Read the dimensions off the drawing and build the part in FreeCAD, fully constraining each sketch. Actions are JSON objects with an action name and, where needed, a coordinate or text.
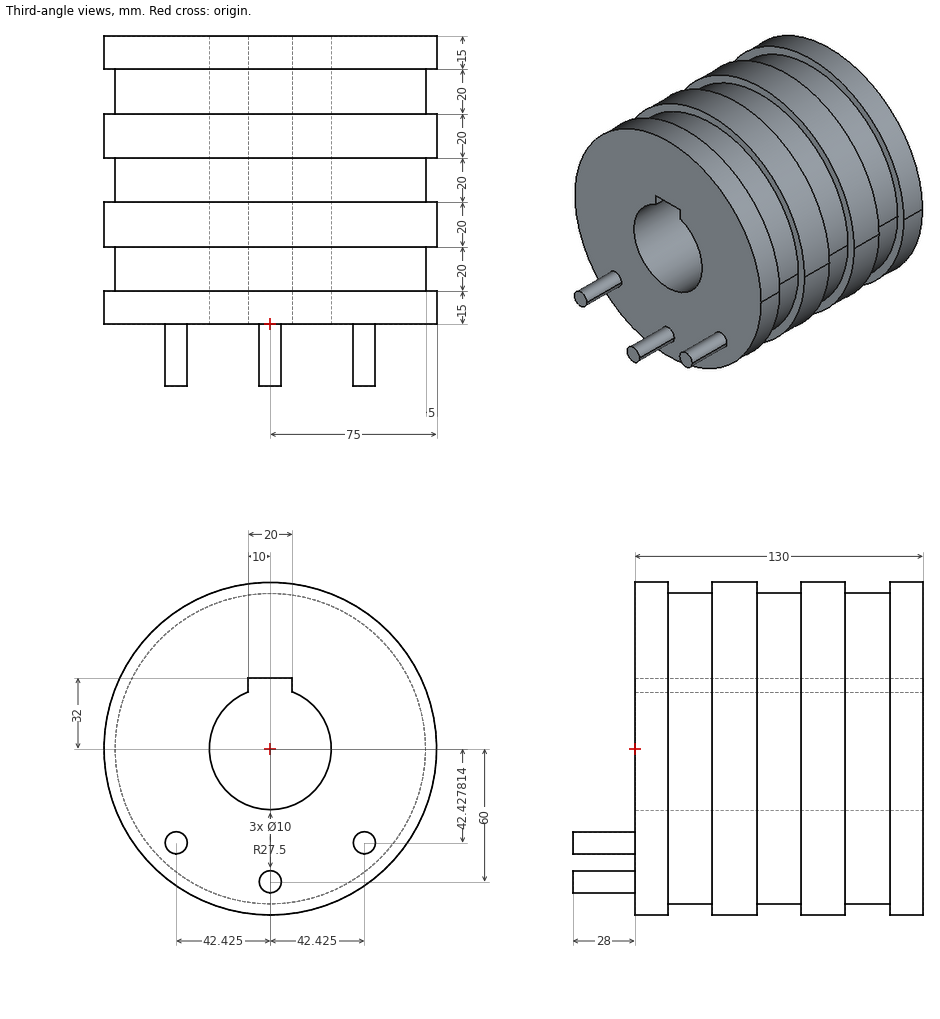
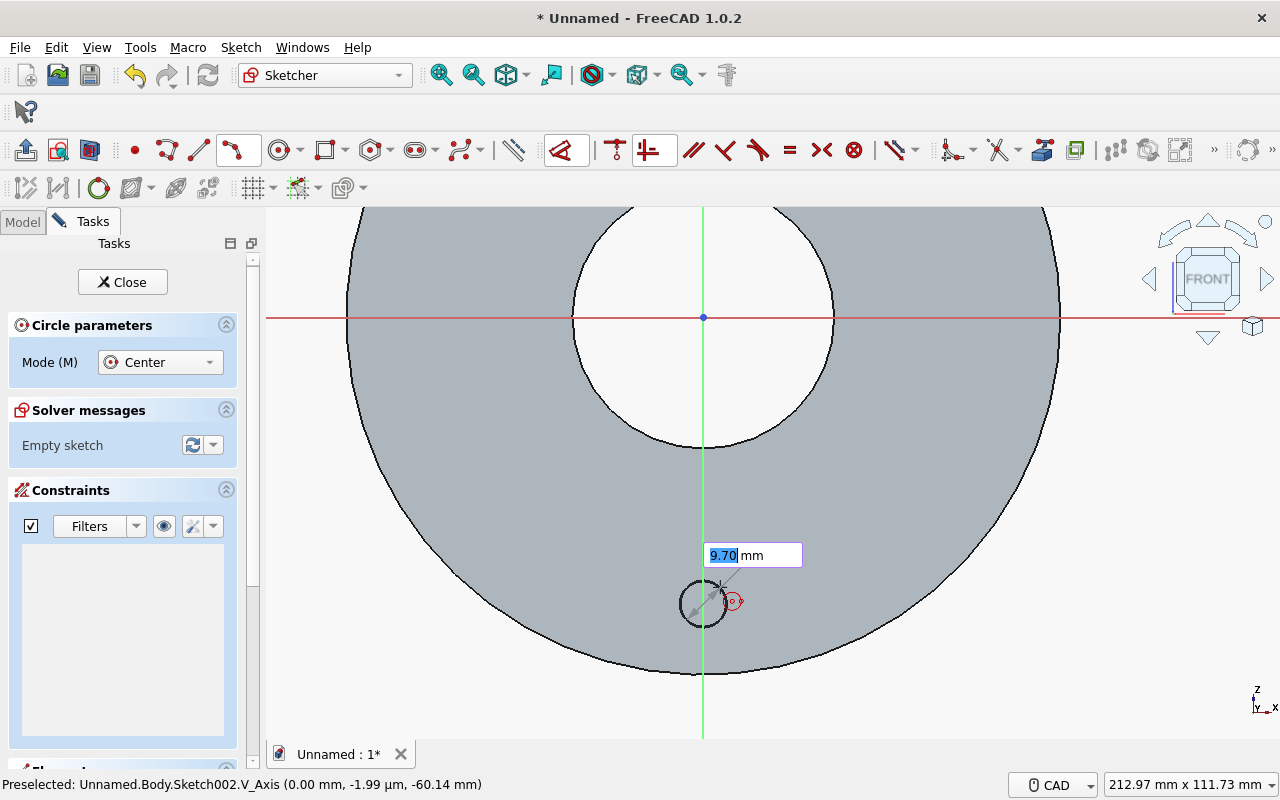
{"action": "type", "text": "10"}
{"action": "key", "text": "Return"}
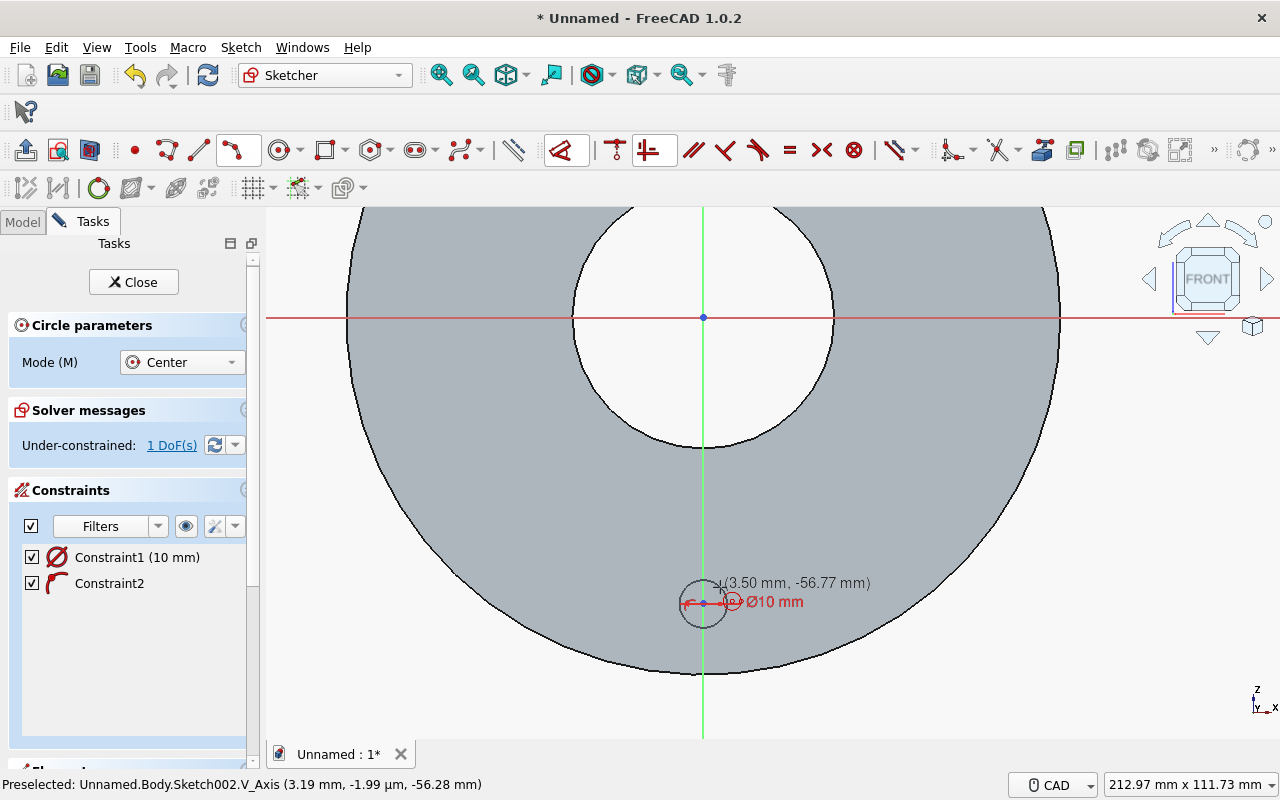
{"action": "left_click", "coordinate": [905, 520]}
{"action": "mouse_move", "coordinate": [922, 503]}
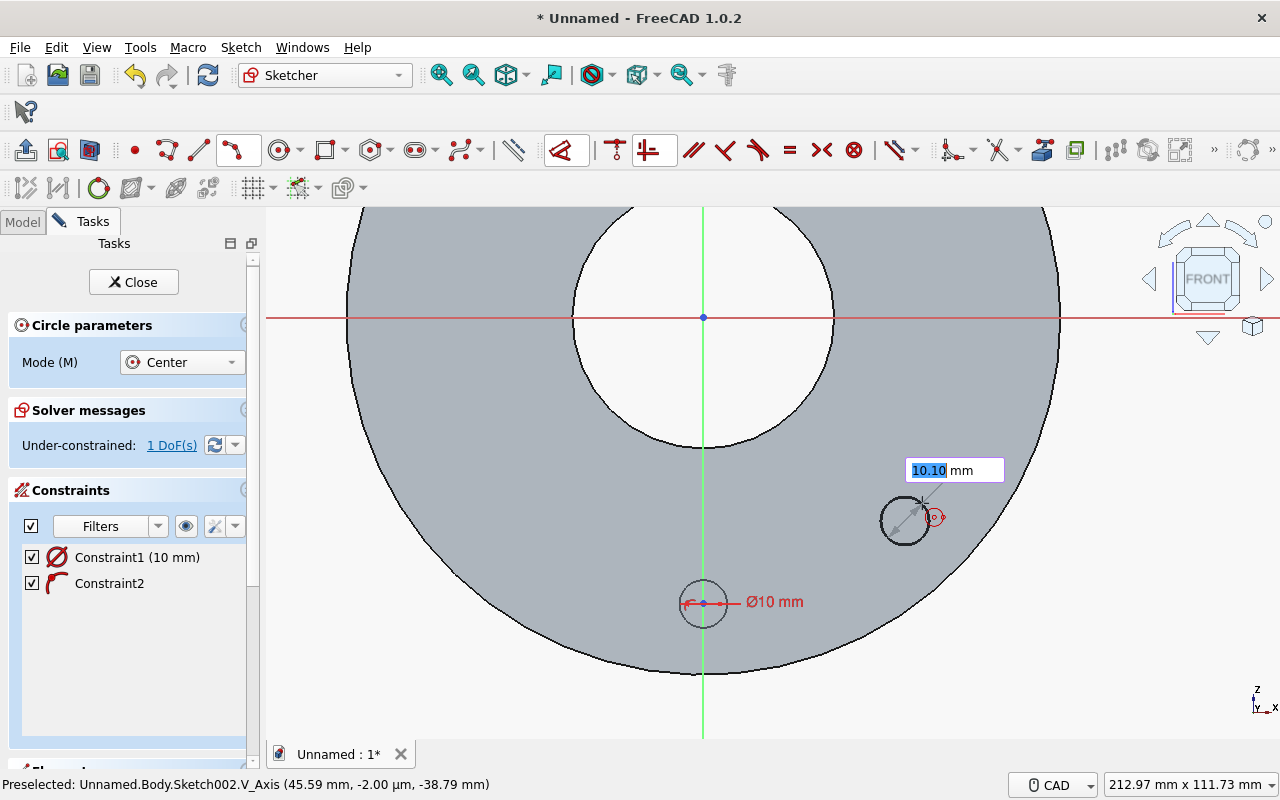
{"action": "type", "text": "10"}
{"action": "key", "text": "Return"}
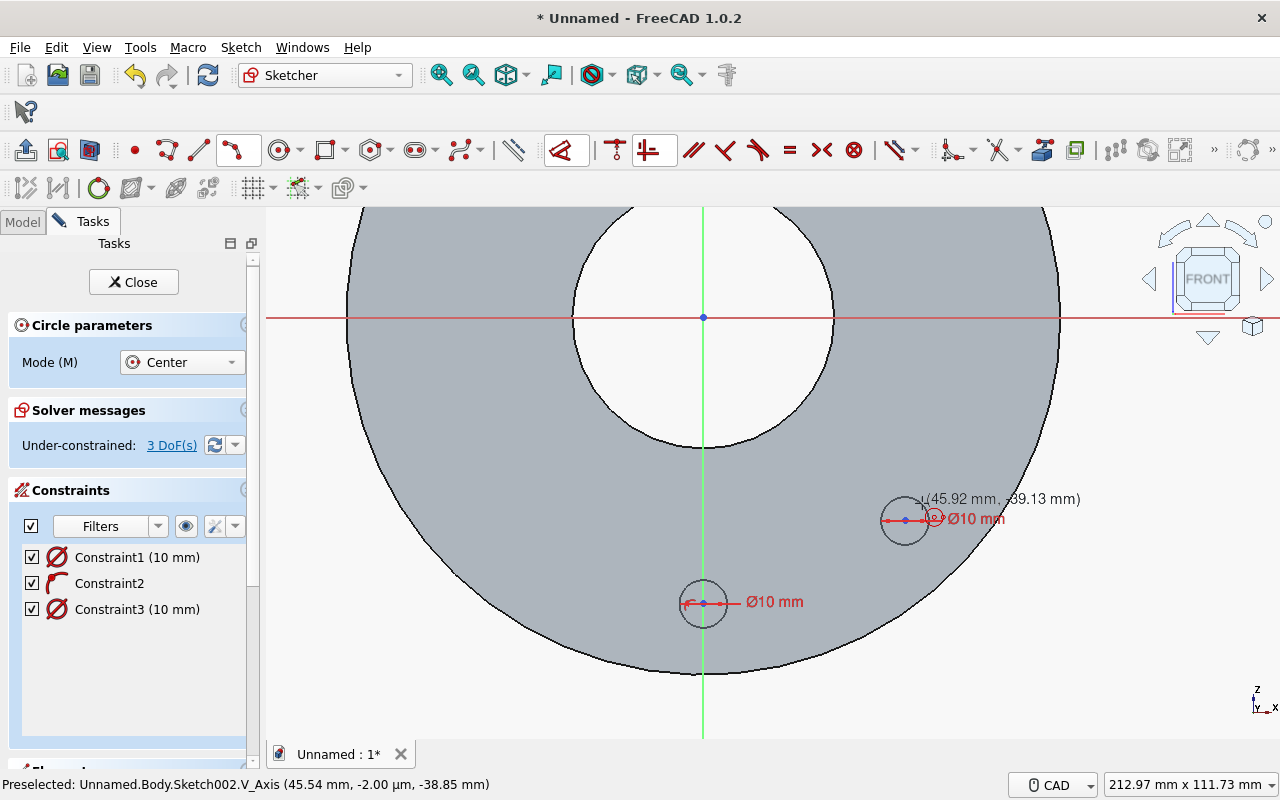
{"action": "left_click", "coordinate": [501, 520]}
{"action": "mouse_move", "coordinate": [518, 503]}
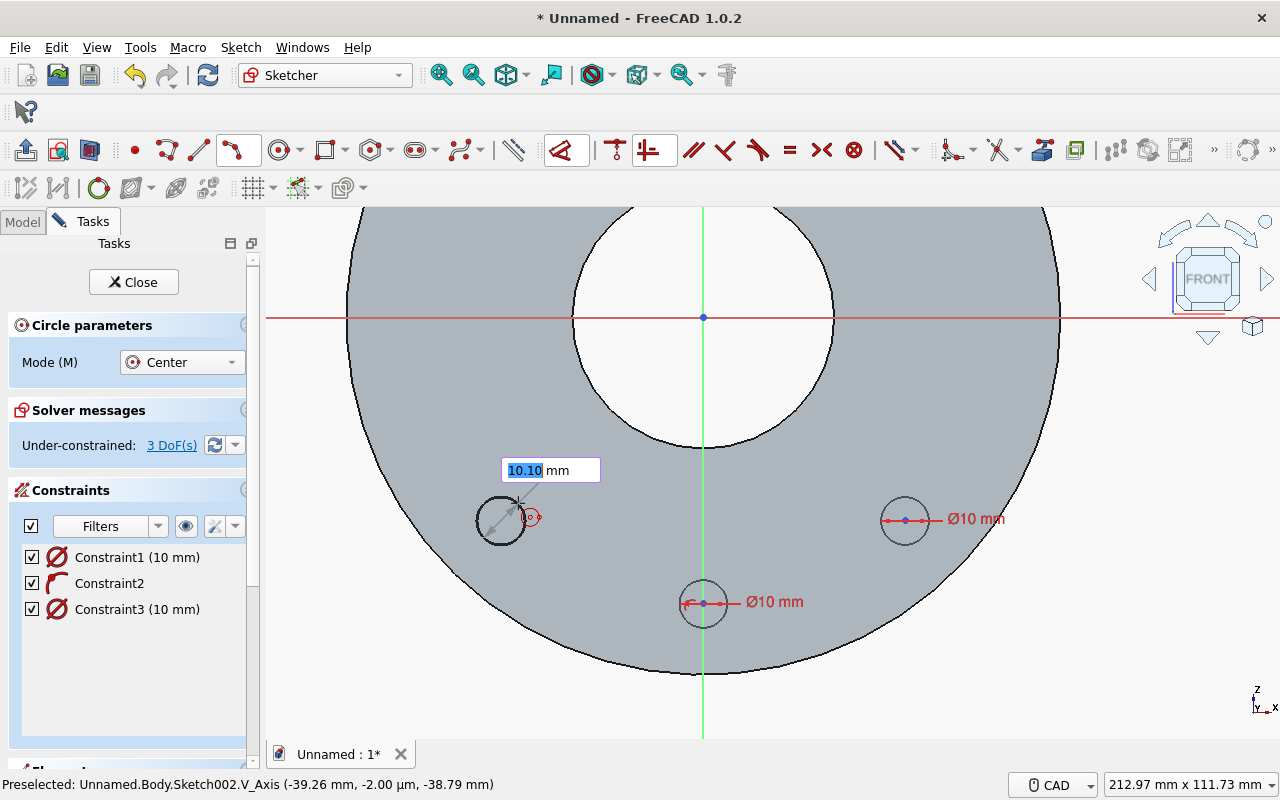
{"action": "type", "text": "10"}
{"action": "key", "text": "Return"}
{"action": "key", "text": "Escape"}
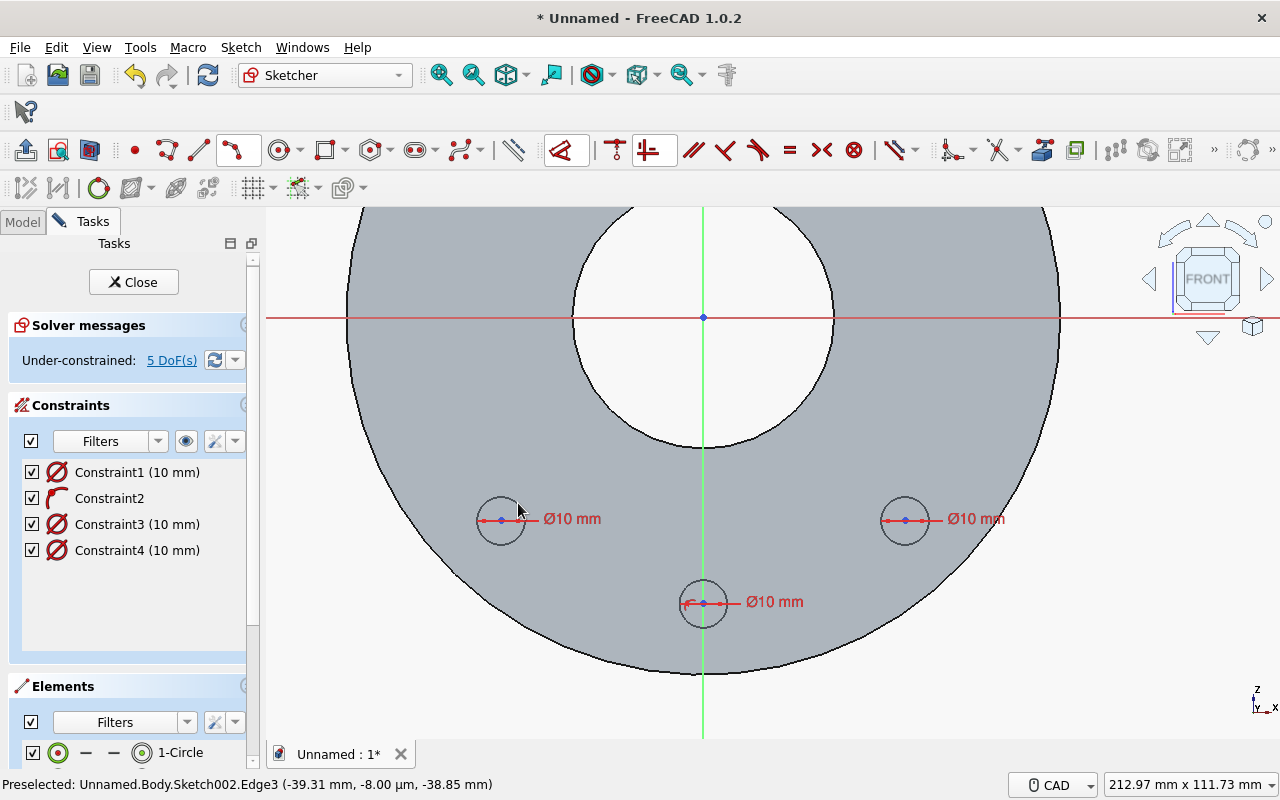
{"action": "left_click", "coordinate": [905, 521]}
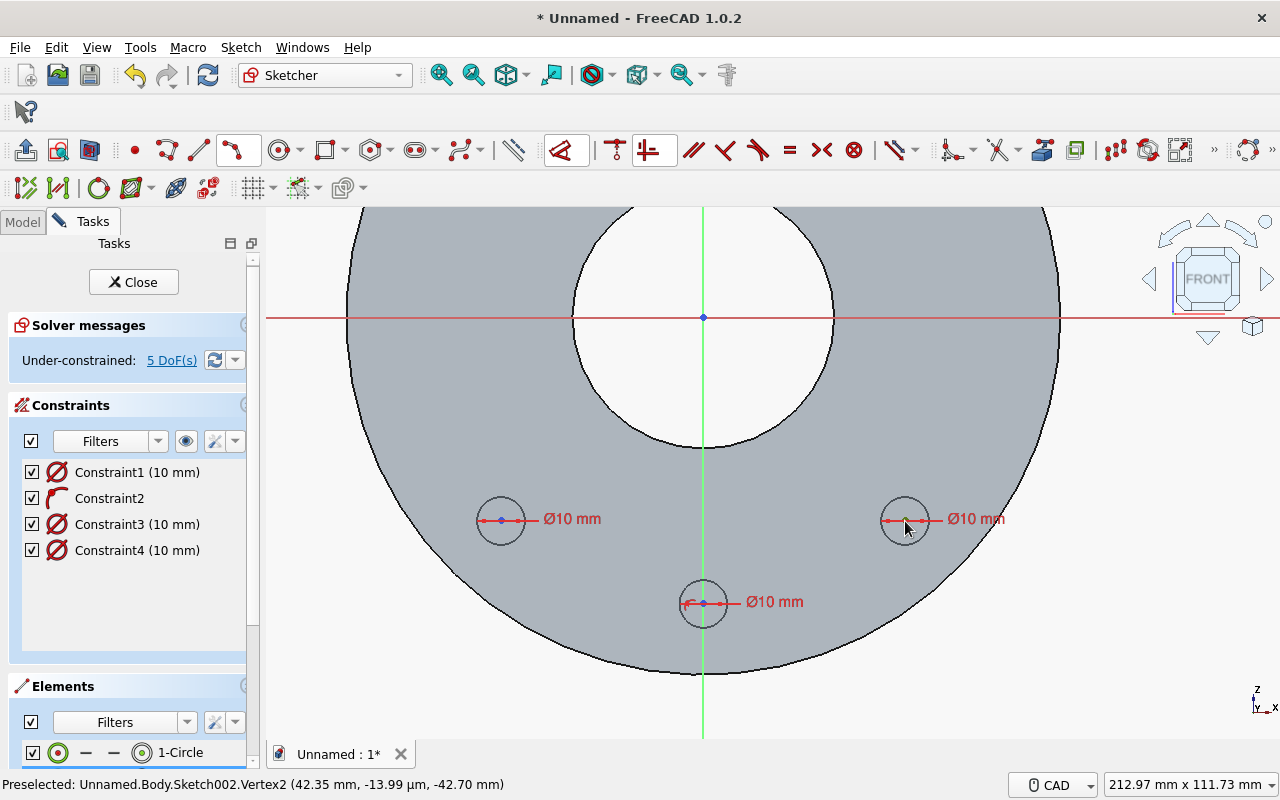
{"action": "left_click", "coordinate": [501, 521]}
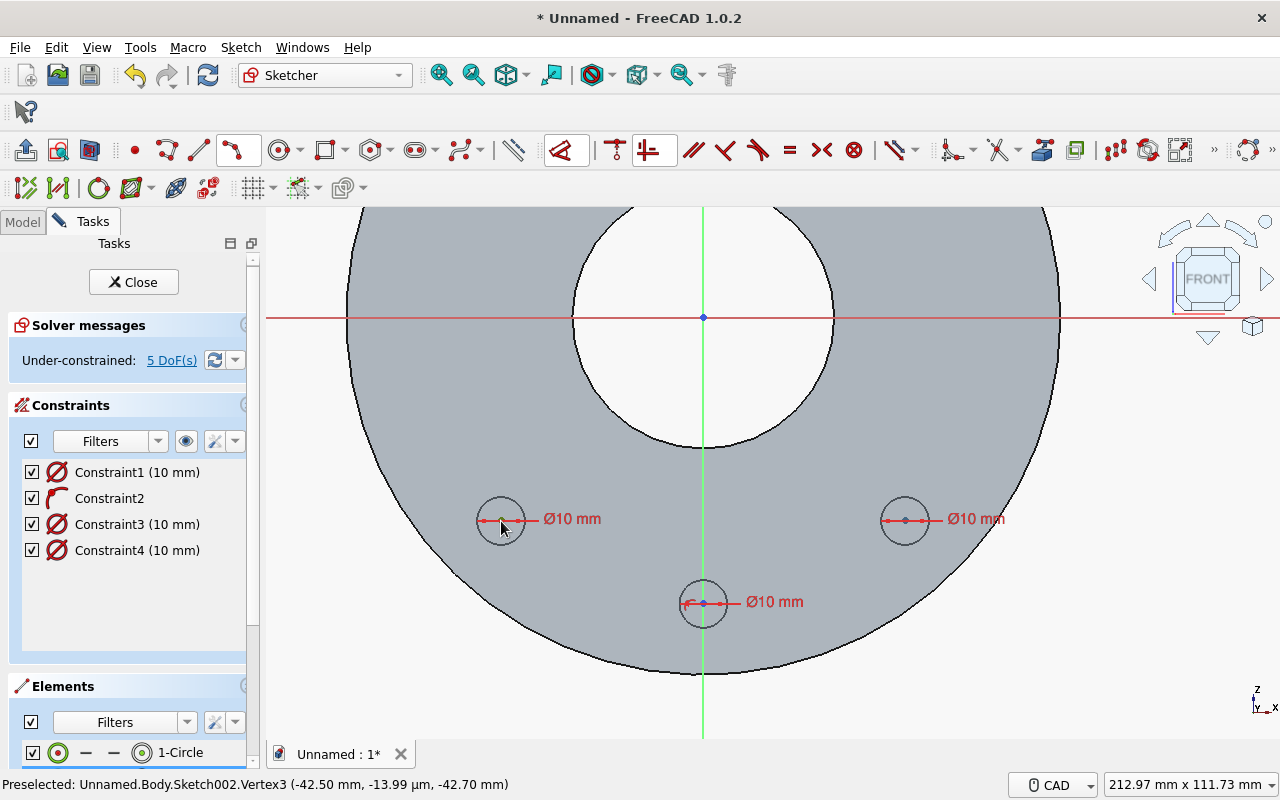
{"action": "key", "text": "h"}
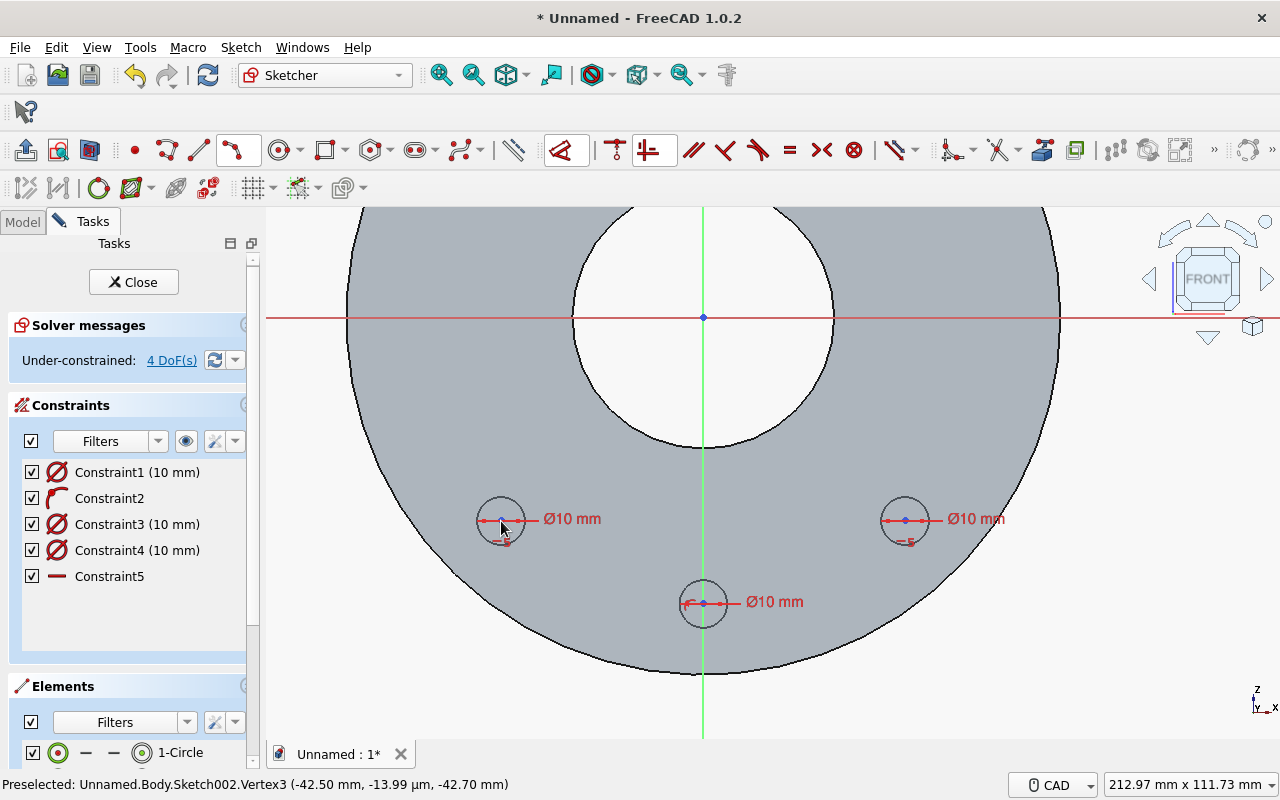
{"action": "left_click", "coordinate": [703, 604]}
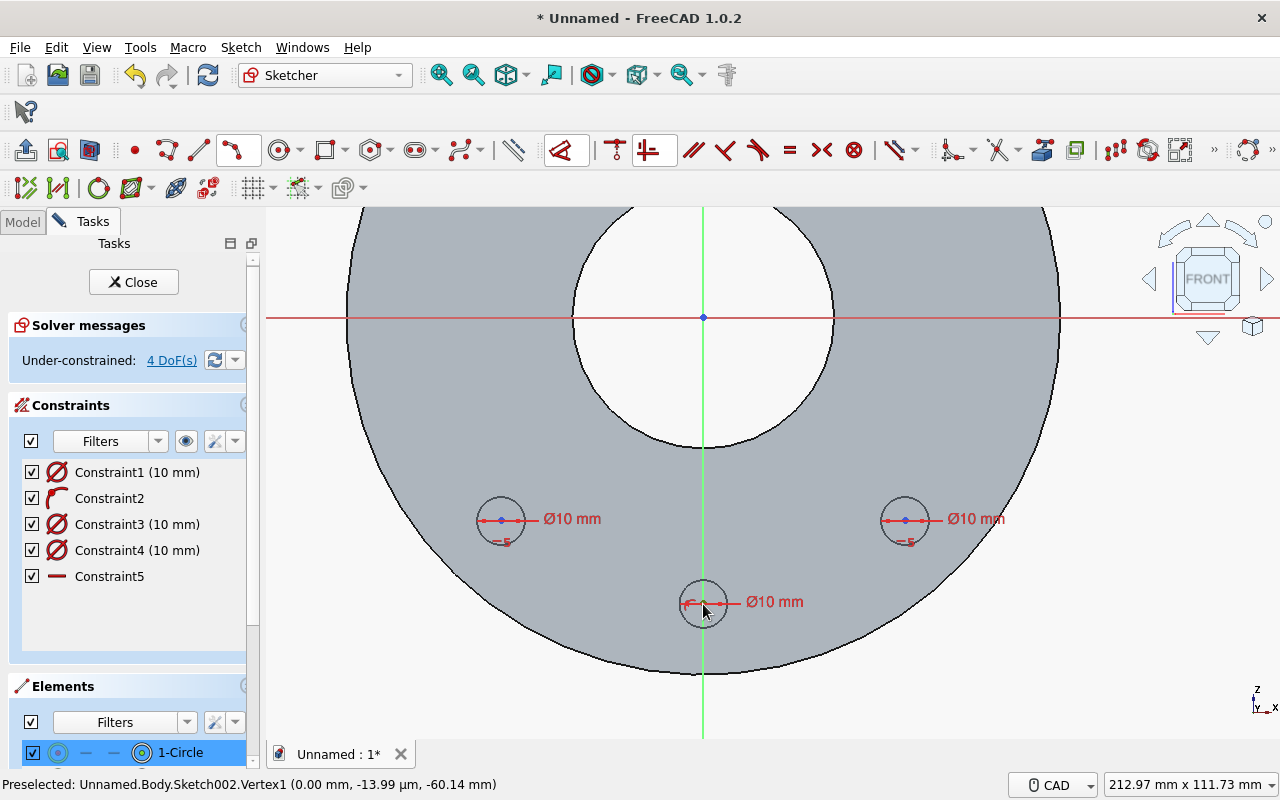
{"action": "key", "text": "i"}